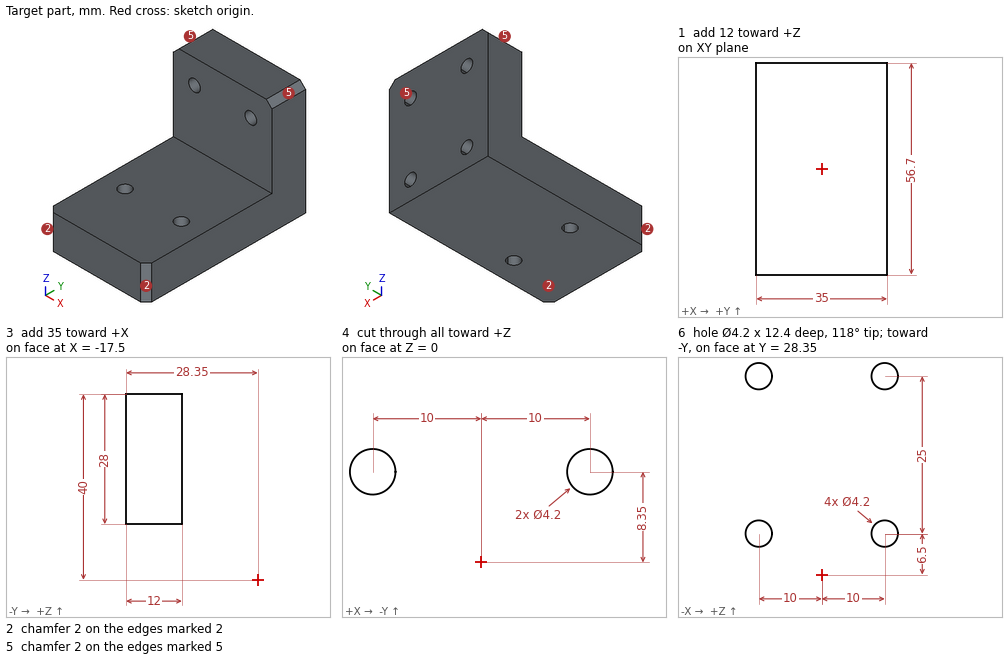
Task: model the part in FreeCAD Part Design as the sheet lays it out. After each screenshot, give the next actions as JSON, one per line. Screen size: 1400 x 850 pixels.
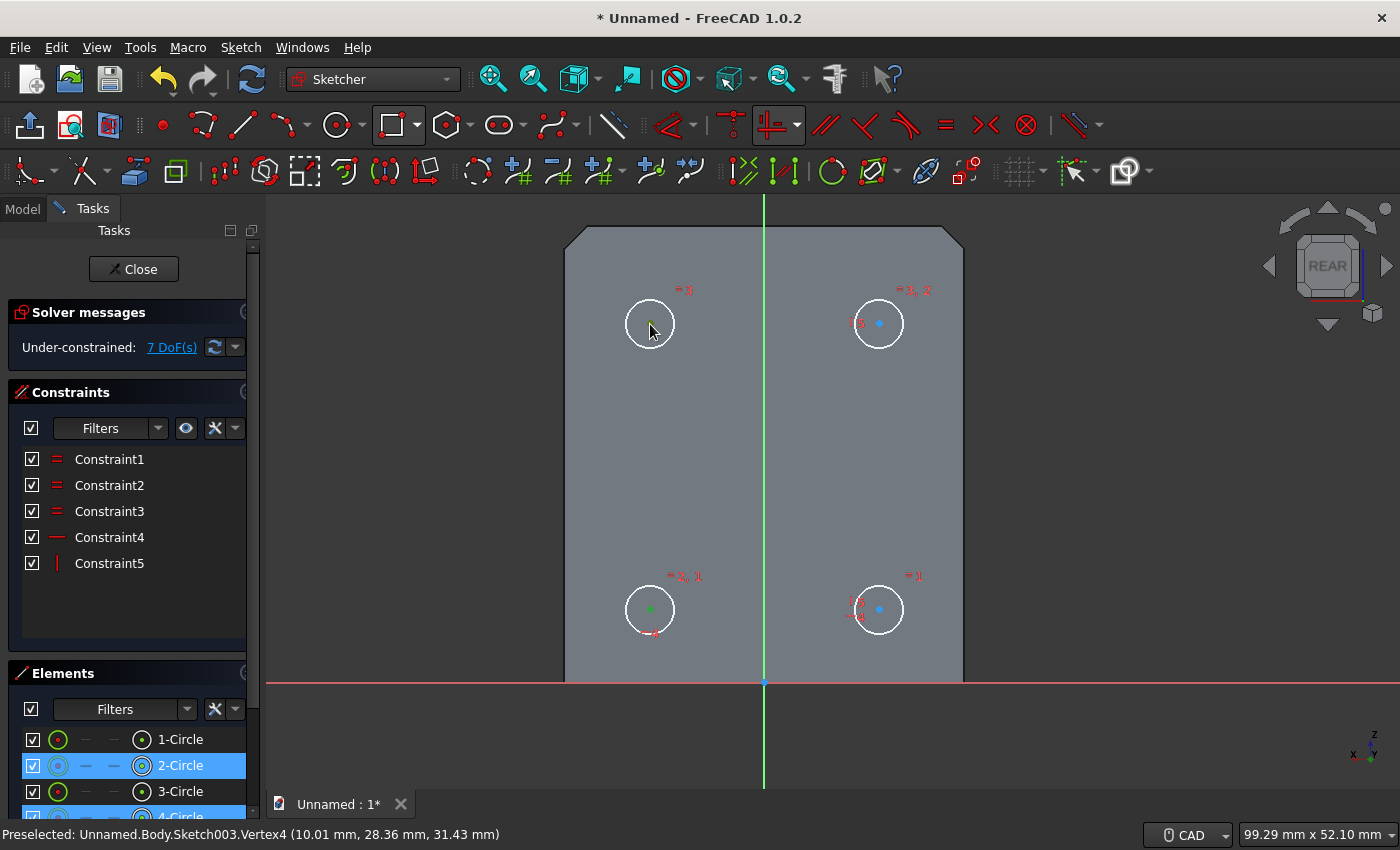
{"action": "key", "text": "v"}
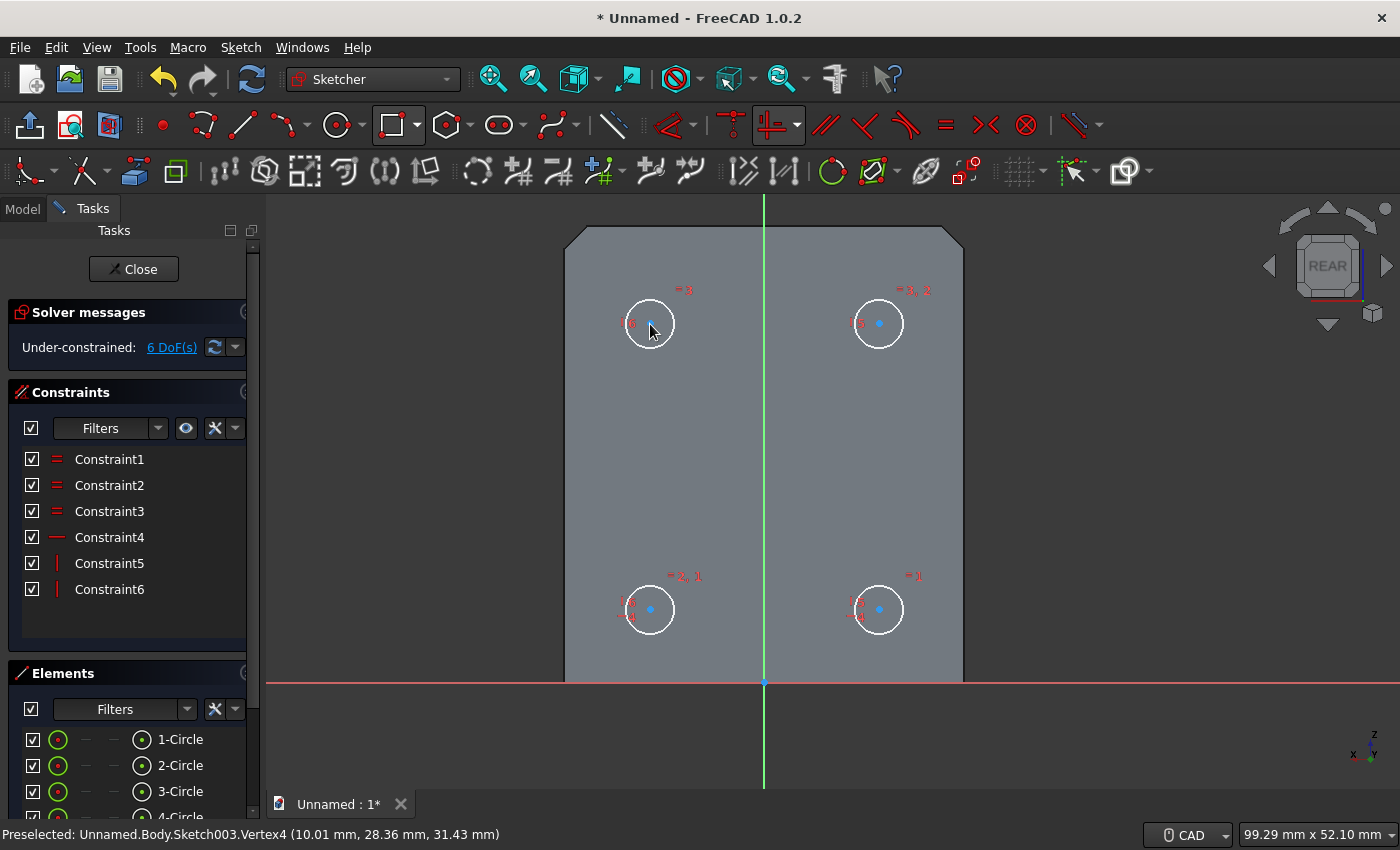
{"action": "left_click", "coordinate": [879, 324]}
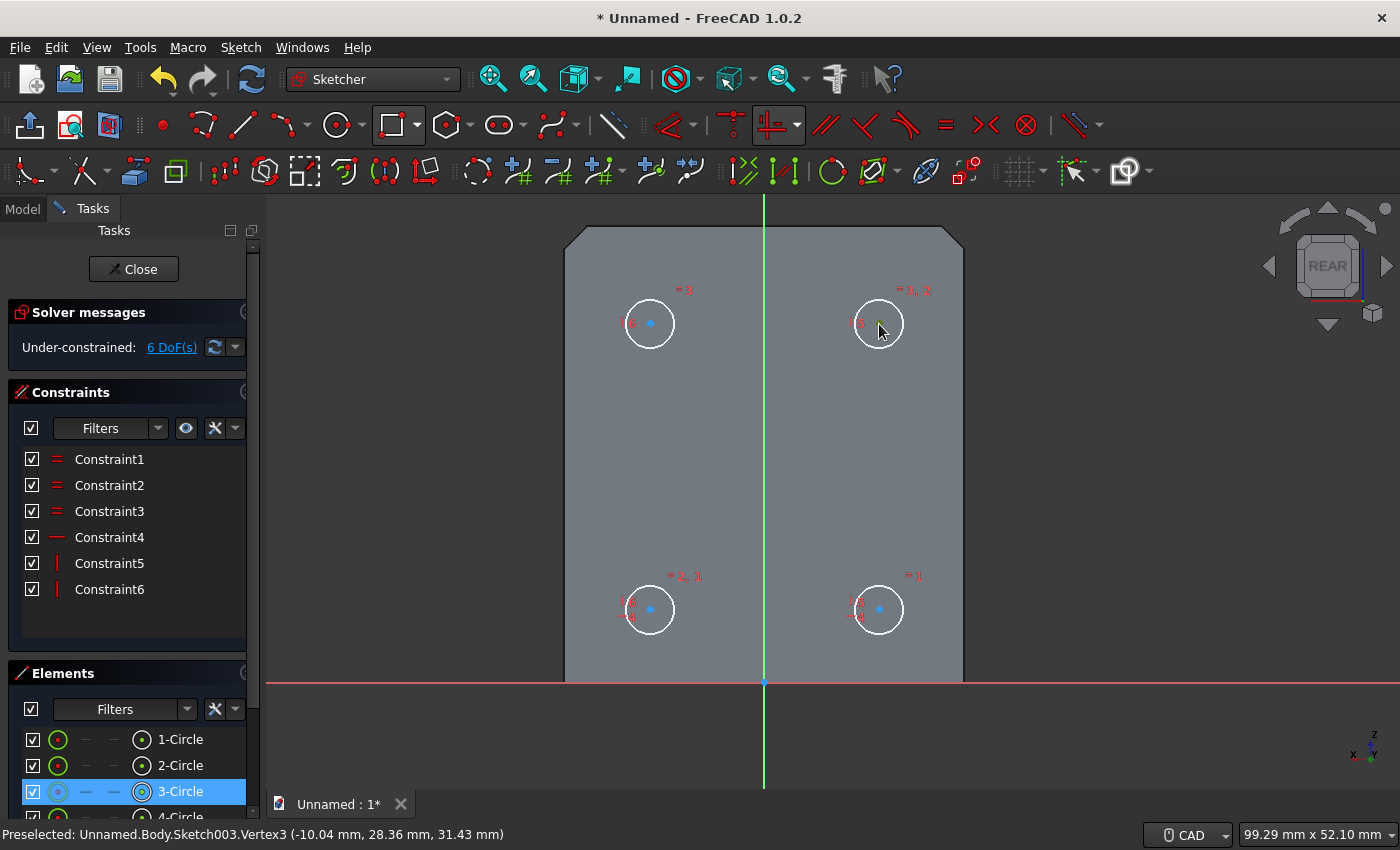
{"action": "left_click", "coordinate": [650, 324]}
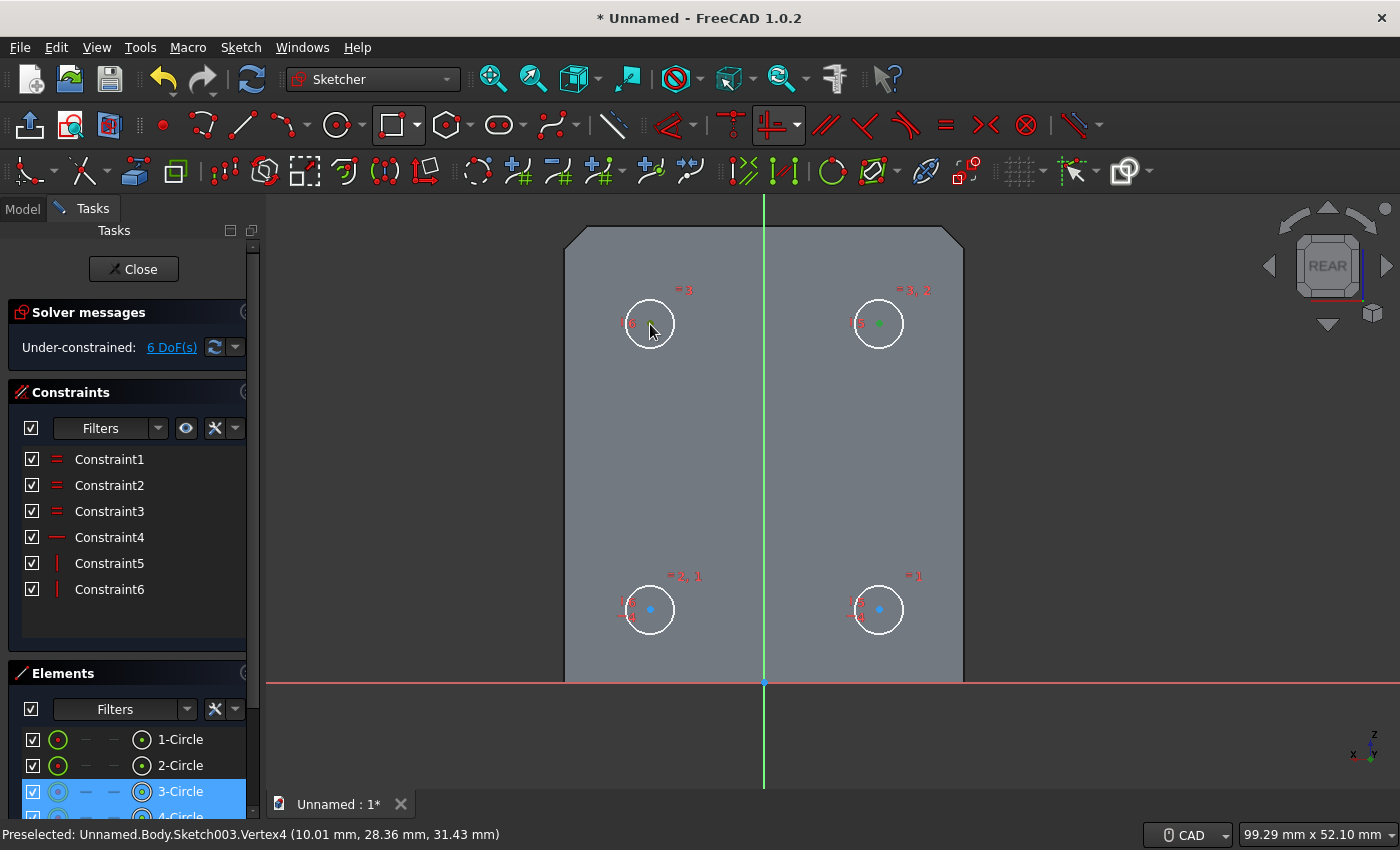
{"action": "key", "text": "h"}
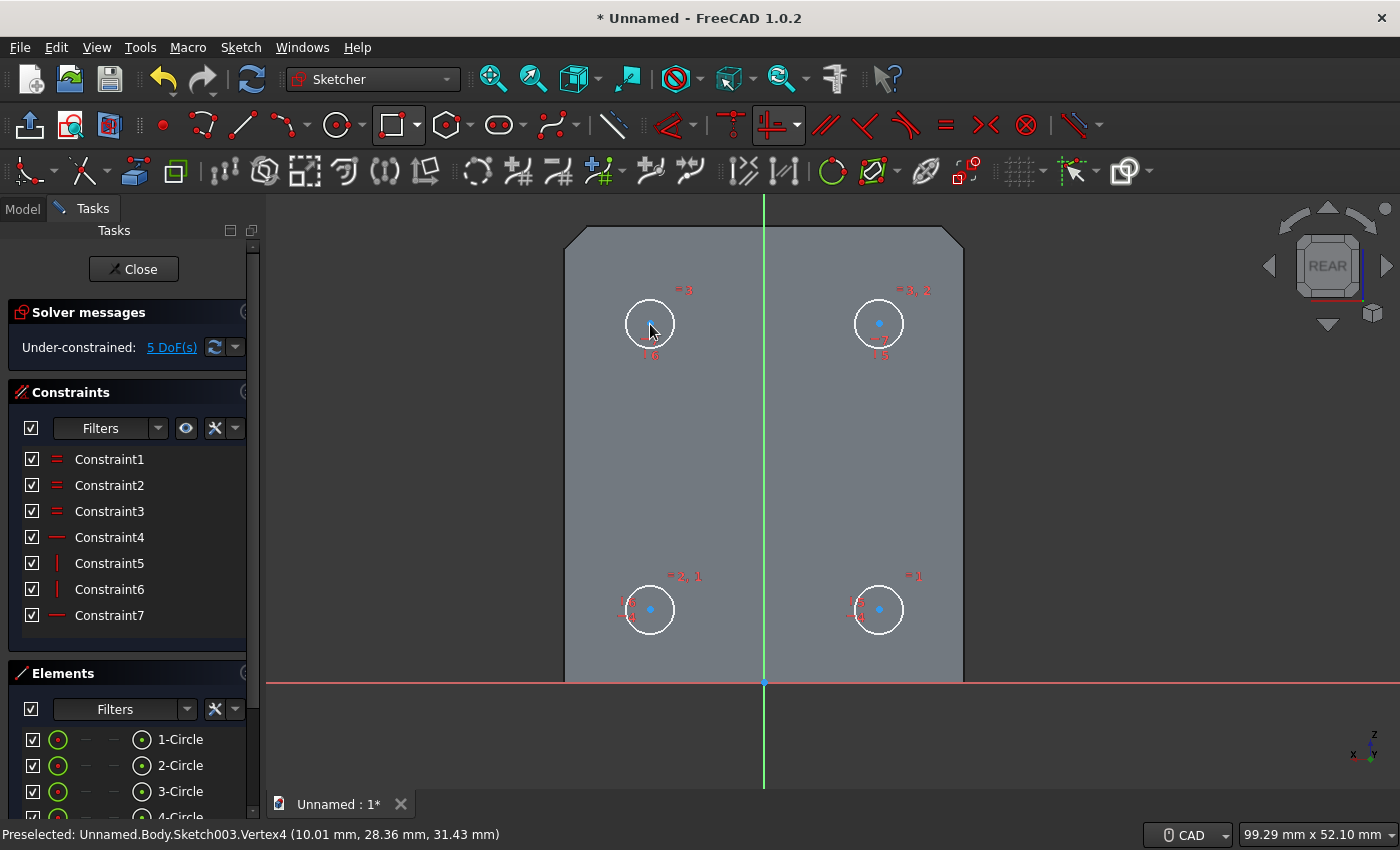
{"action": "left_click", "coordinate": [668, 126]}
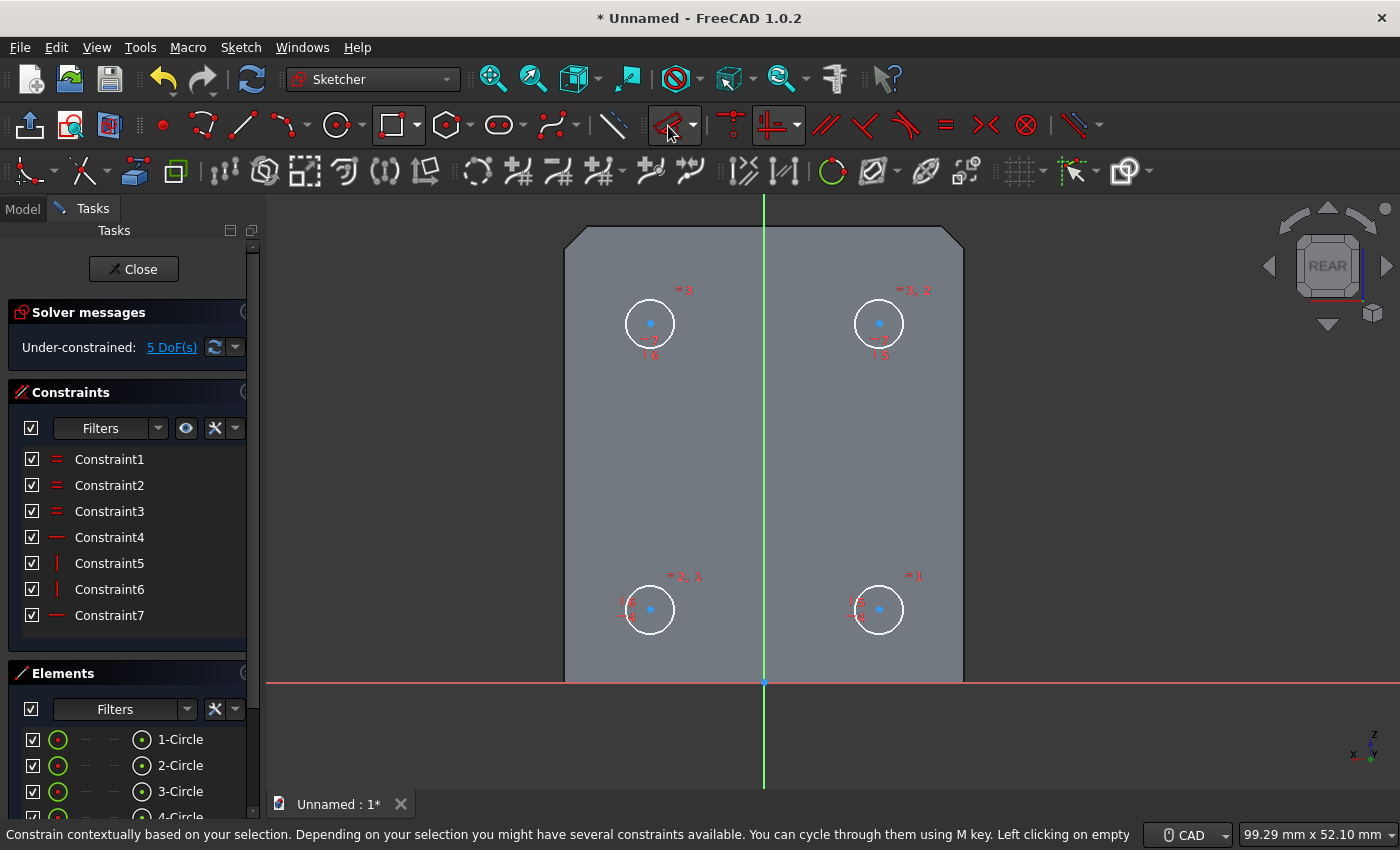
{"action": "left_click", "coordinate": [896, 593]}
{"action": "left_click", "coordinate": [919, 570]}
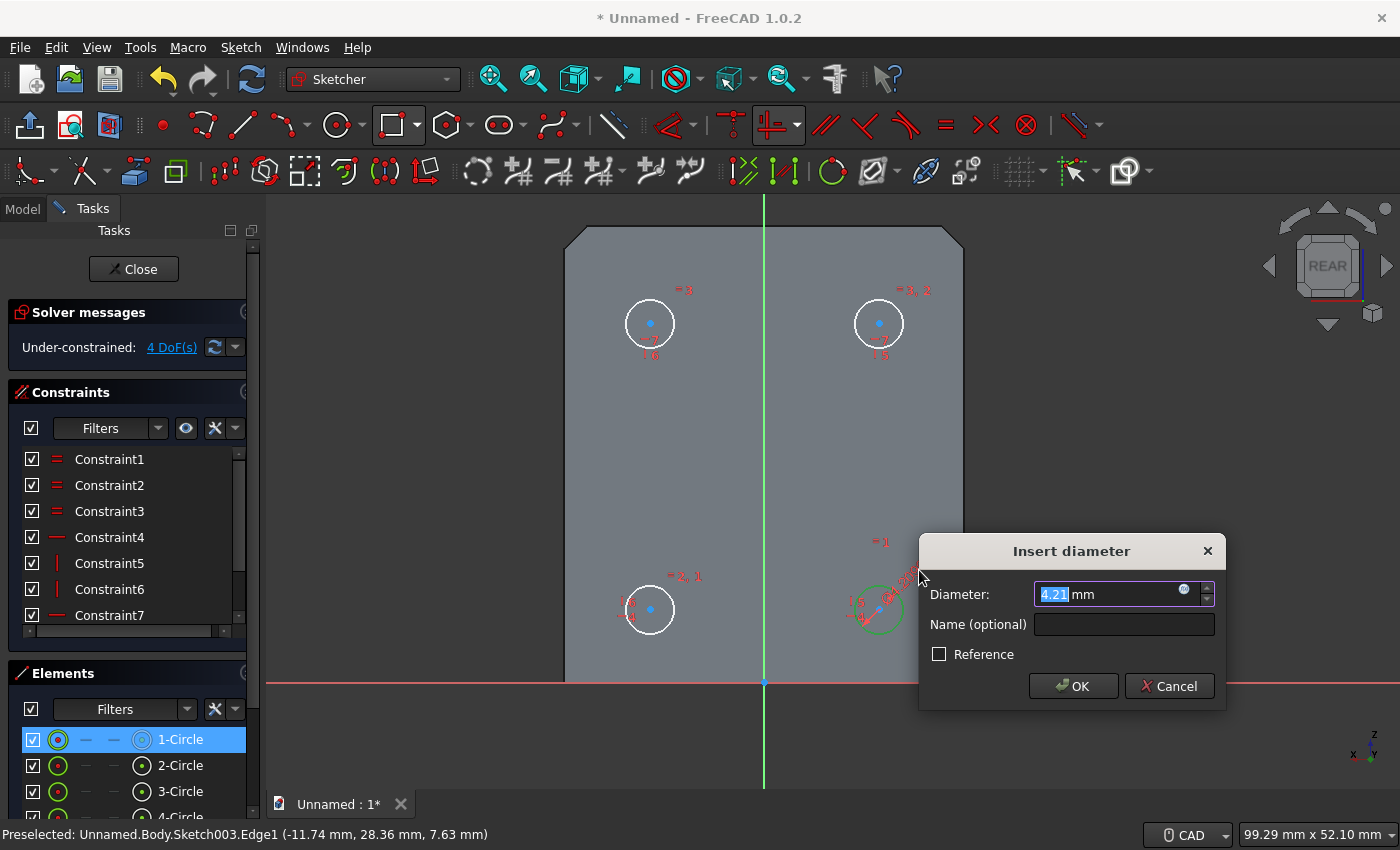
{"action": "type", "text": "4.2"}
{"action": "key", "text": "Return"}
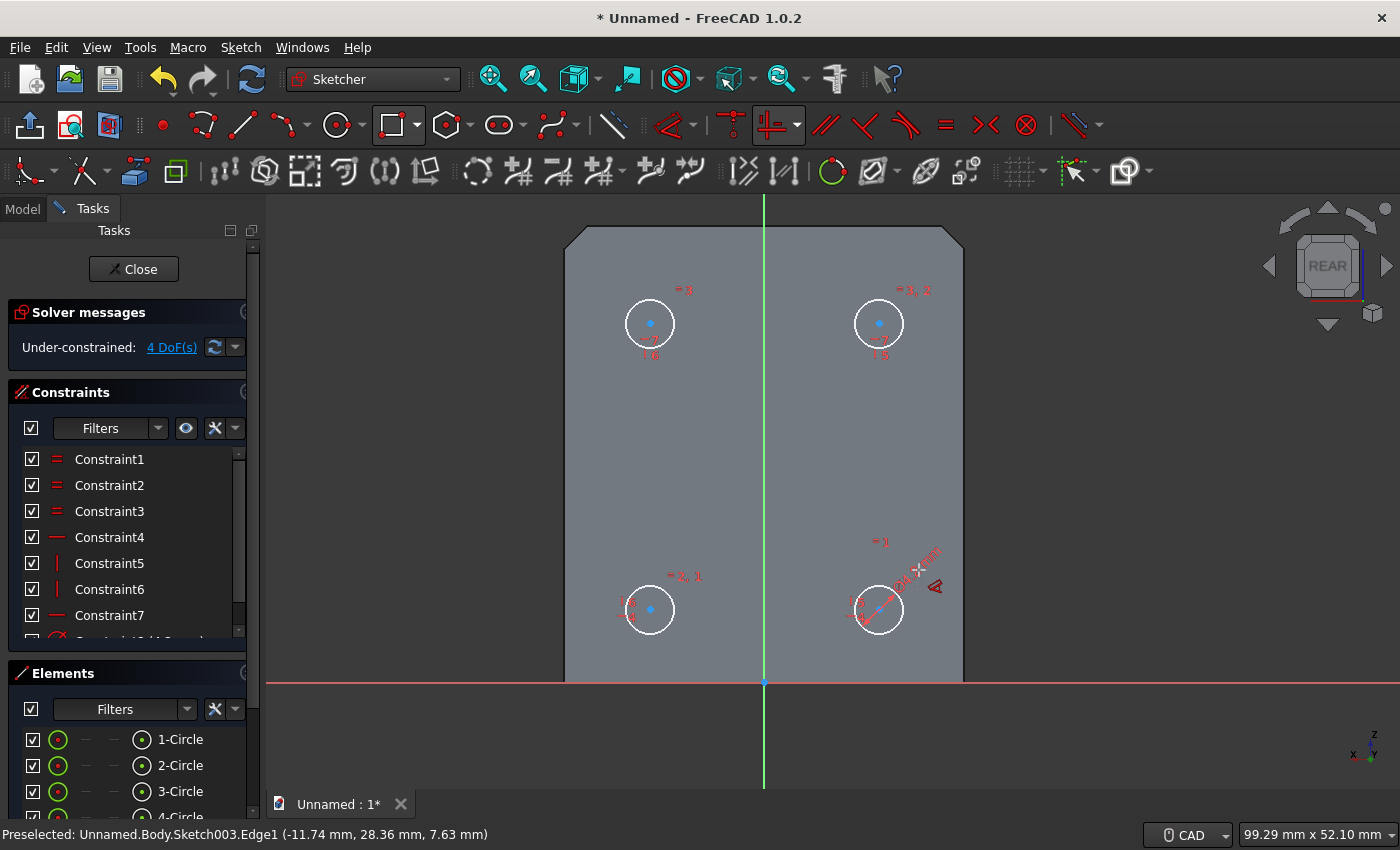
{"action": "left_click", "coordinate": [879, 610]}
{"action": "left_click", "coordinate": [822, 717]}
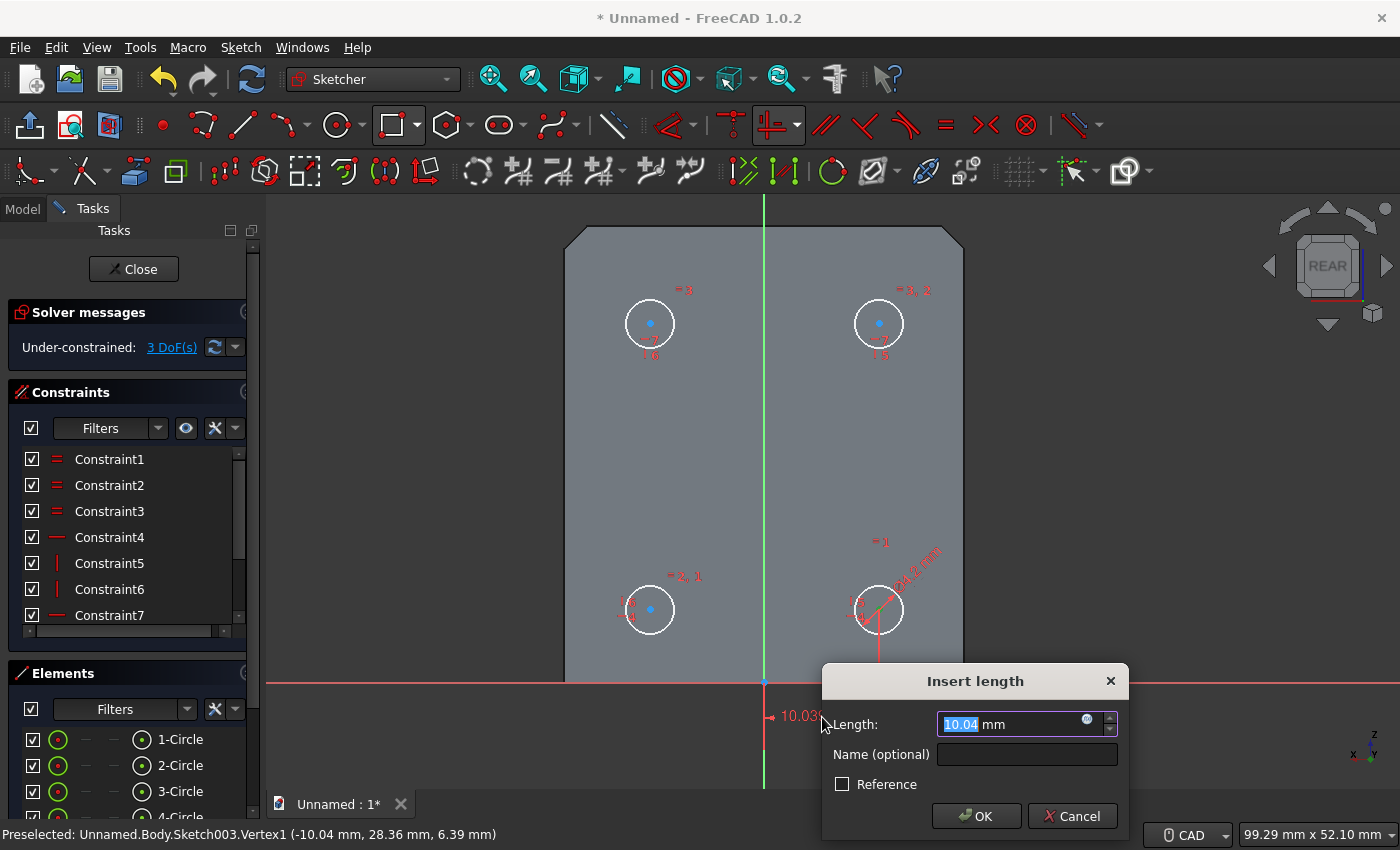
{"action": "type", "text": "10"}
{"action": "key", "text": "Return"}